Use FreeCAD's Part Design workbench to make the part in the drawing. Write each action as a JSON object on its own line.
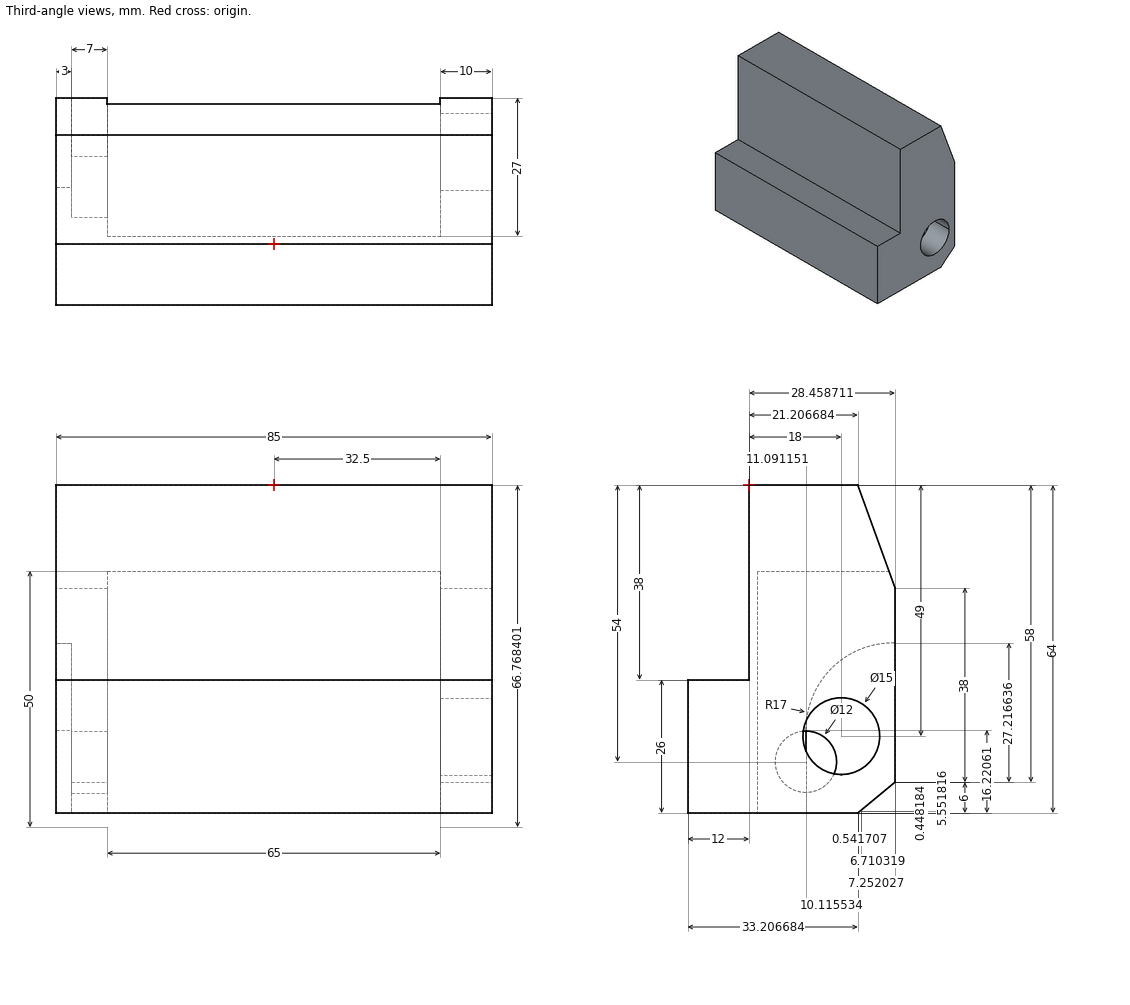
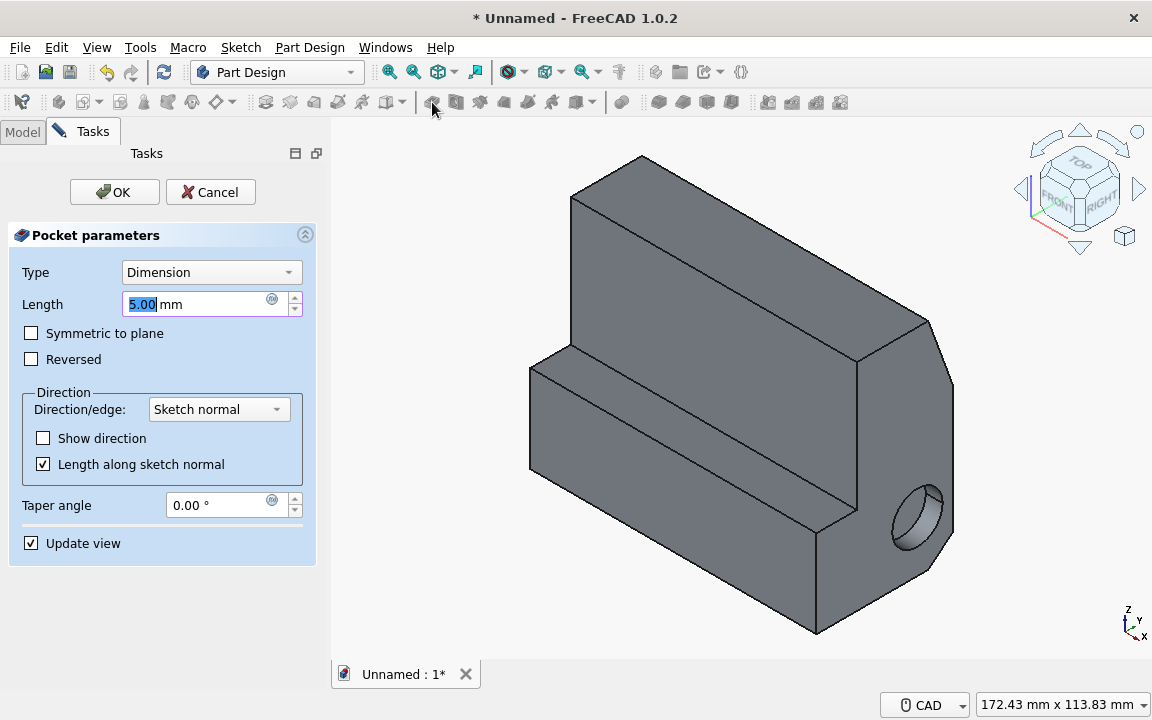
{"action": "type", "text": "10"}
{"action": "key", "text": "Tab"}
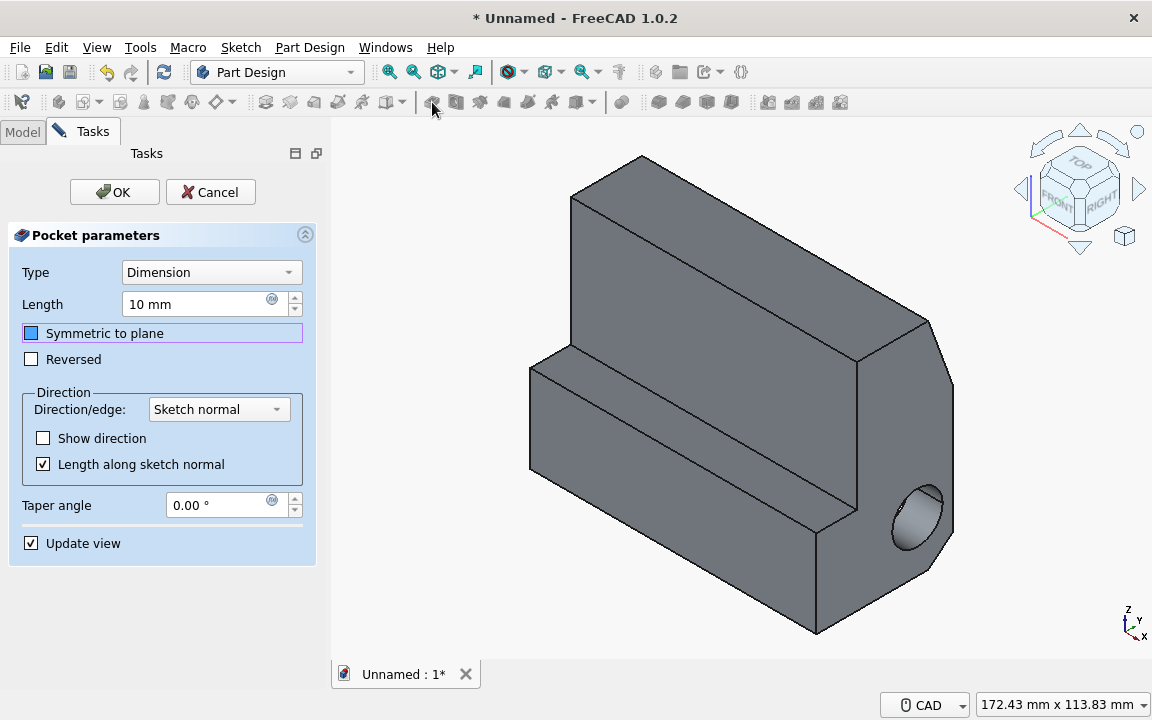
{"action": "left_click", "coordinate": [115, 192]}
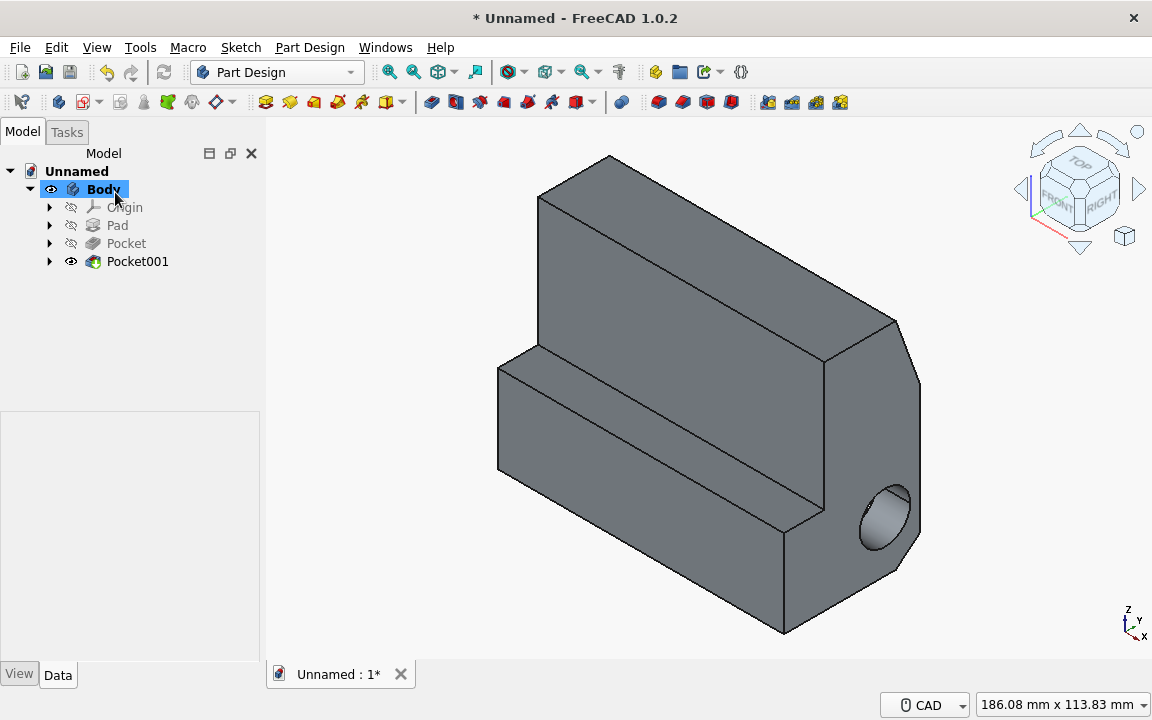
{"action": "key", "text": "6"}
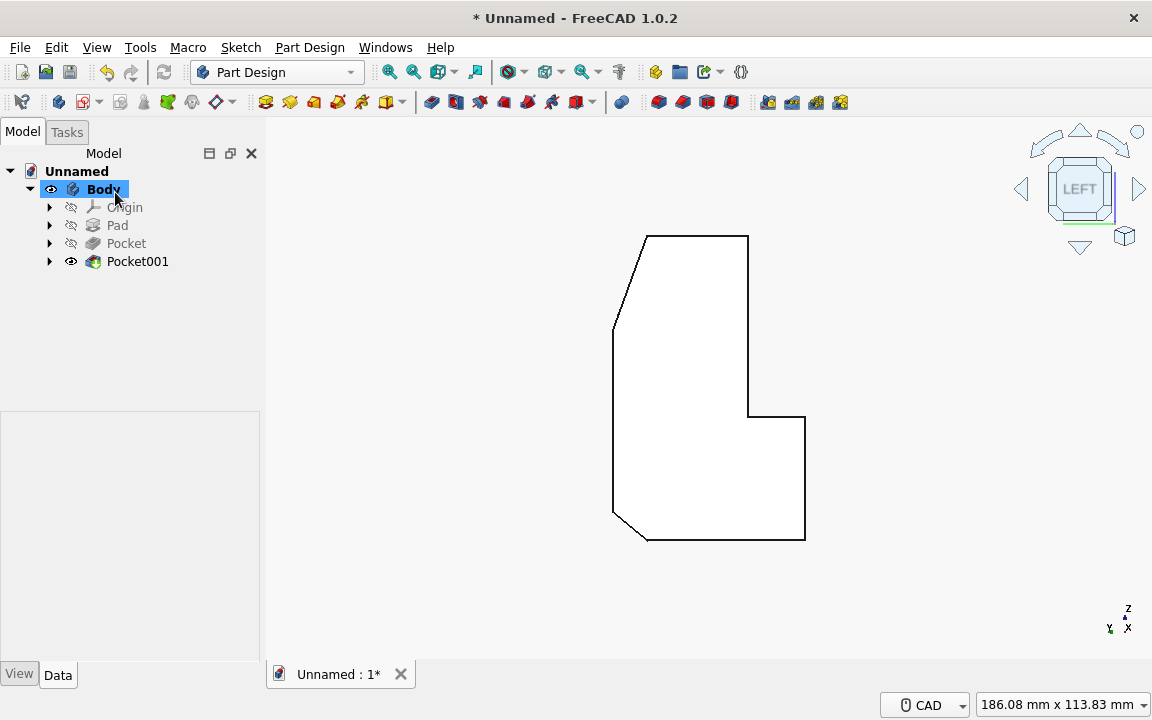
{"action": "left_click", "coordinate": [681, 431]}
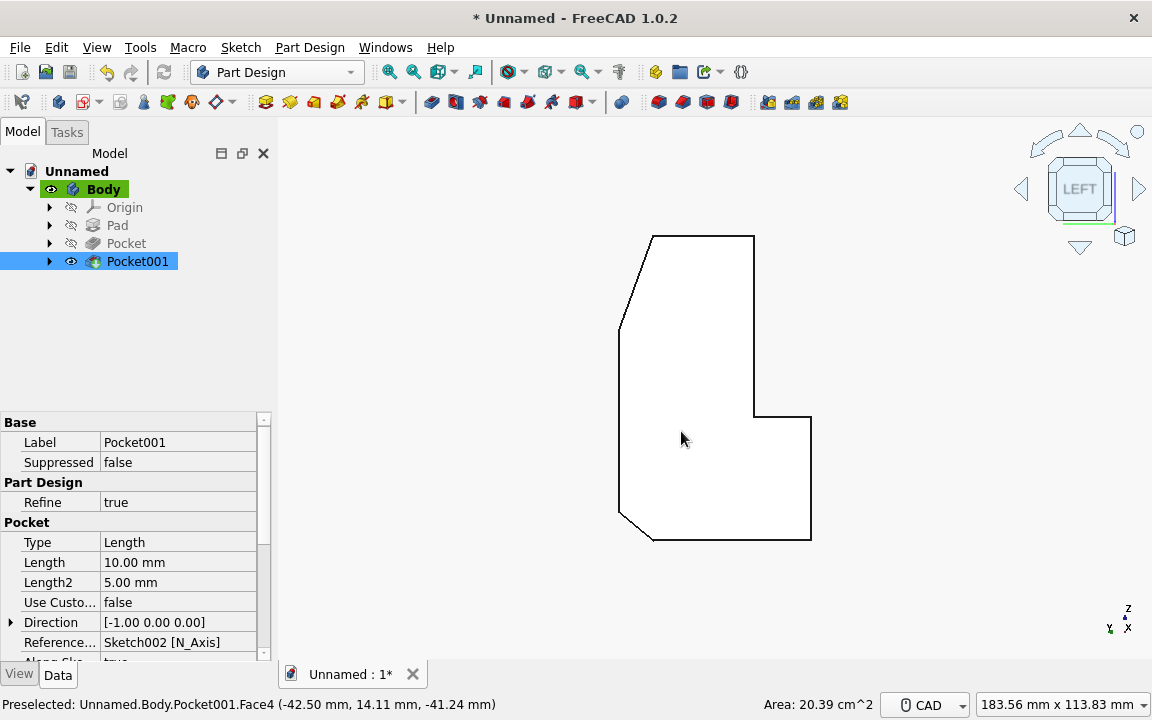
{"action": "left_click", "coordinate": [84, 102]}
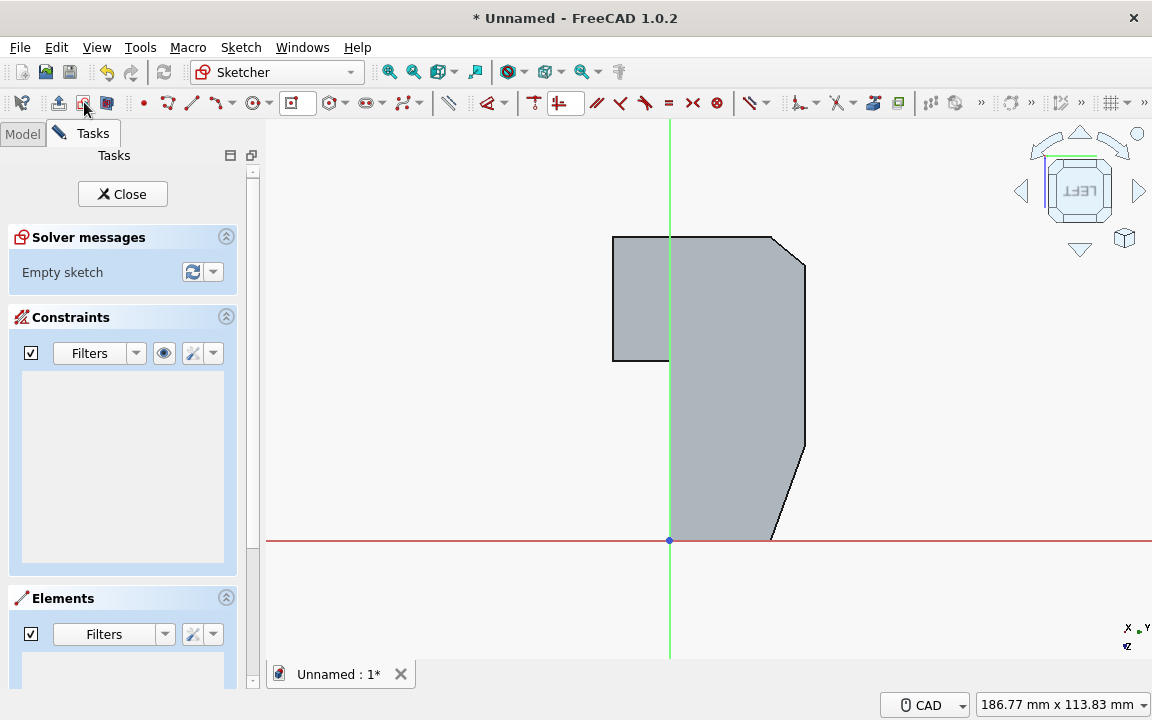
{"action": "left_click", "coordinate": [168, 104]}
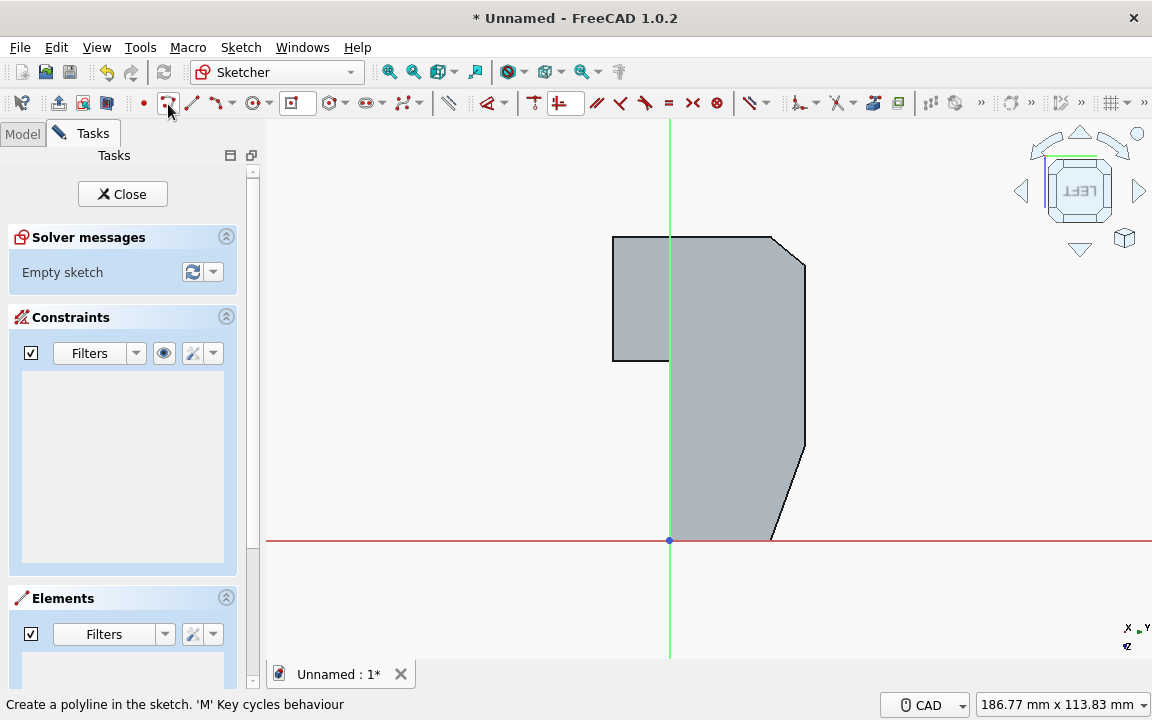
{"action": "left_click", "coordinate": [805, 395]}
{"action": "left_click", "coordinate": [805, 266]}
{"action": "left_click", "coordinate": [773, 239]}
{"action": "right_click", "coordinate": [773, 239]}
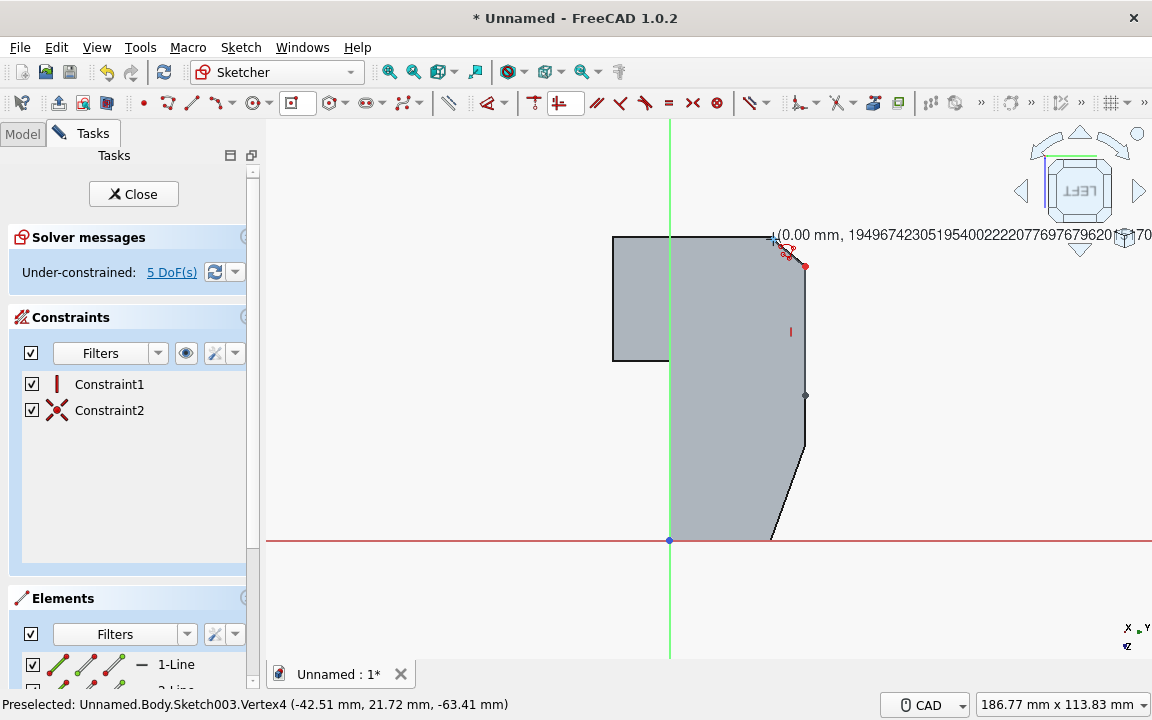
{"action": "left_click", "coordinate": [216, 104]}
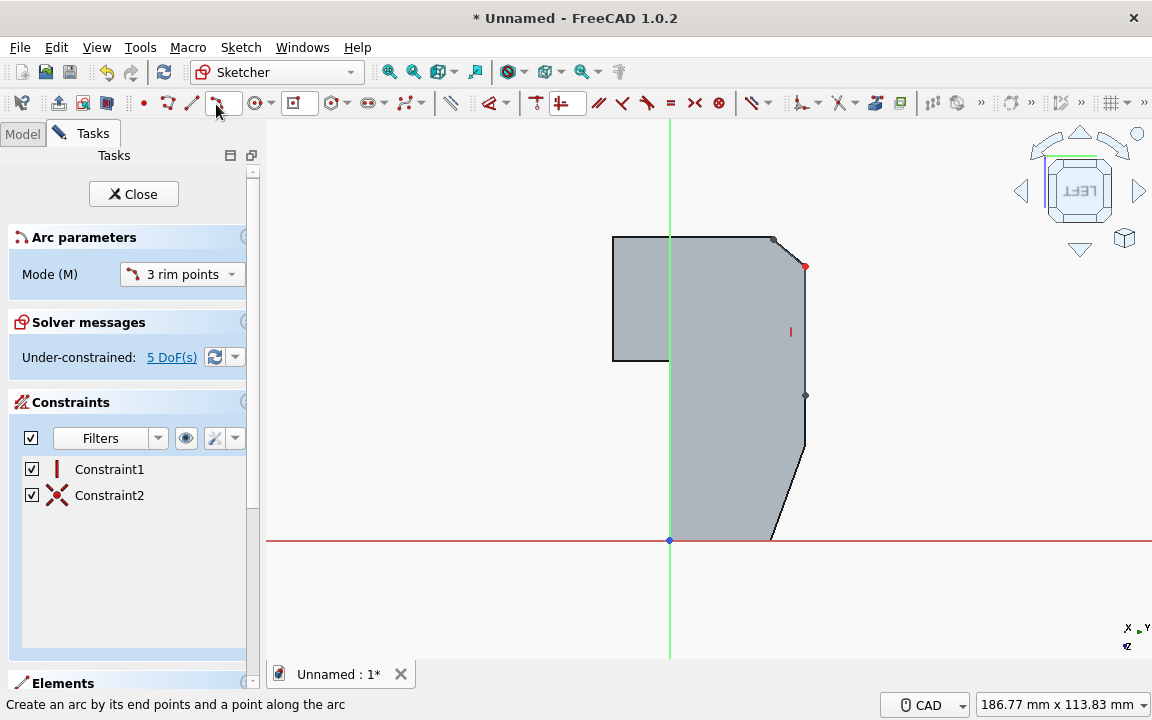
{"action": "left_click", "coordinate": [773, 240]}
{"action": "left_click", "coordinate": [805, 396]}
{"action": "left_click", "coordinate": [724, 330]}
{"action": "key", "text": "Escape"}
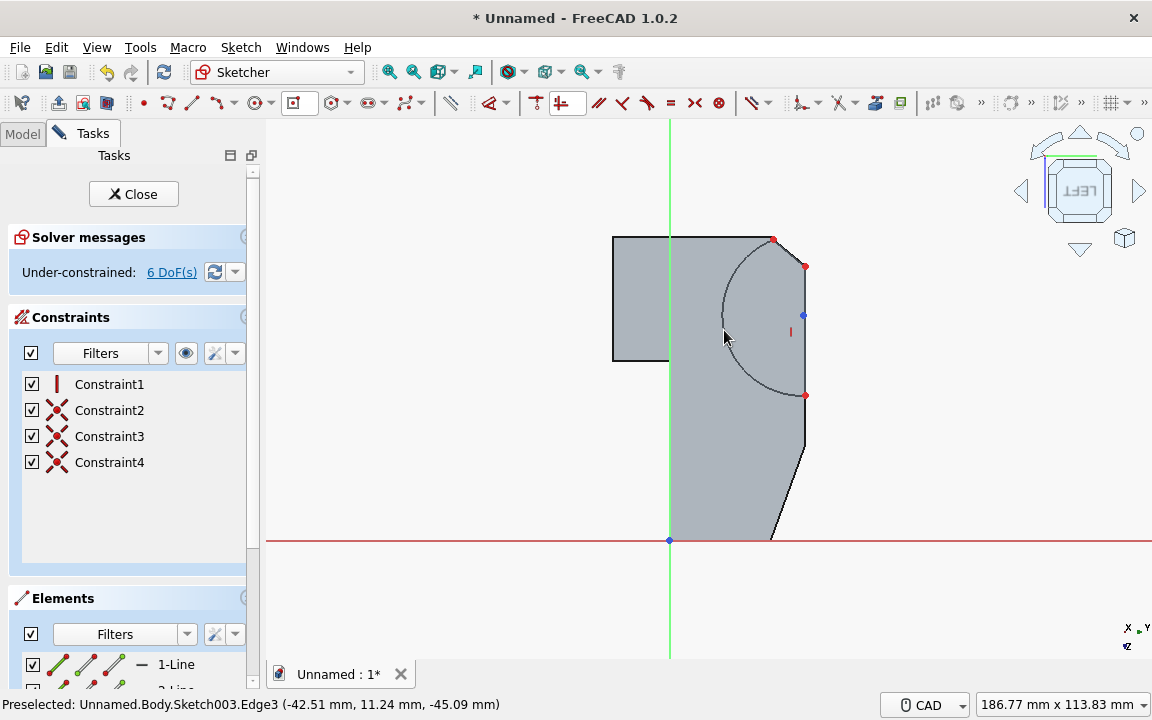
{"action": "left_click", "coordinate": [490, 104]}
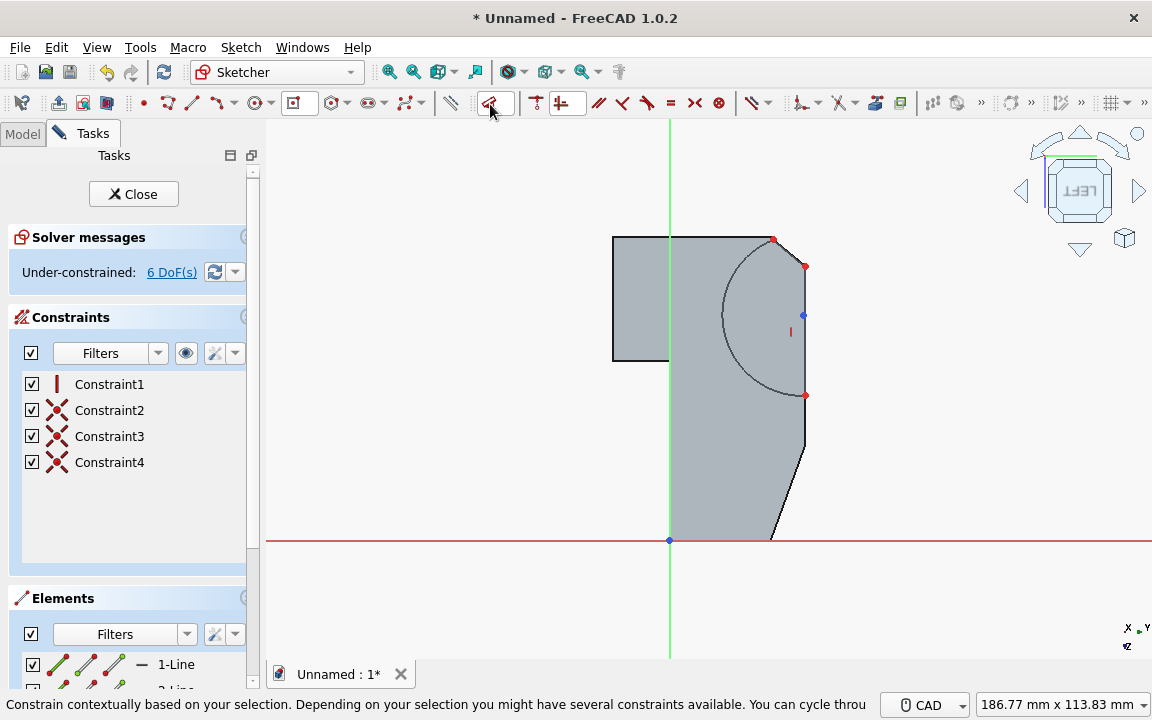
{"action": "left_click", "coordinate": [727, 287]}
{"action": "left_click", "coordinate": [697, 276]}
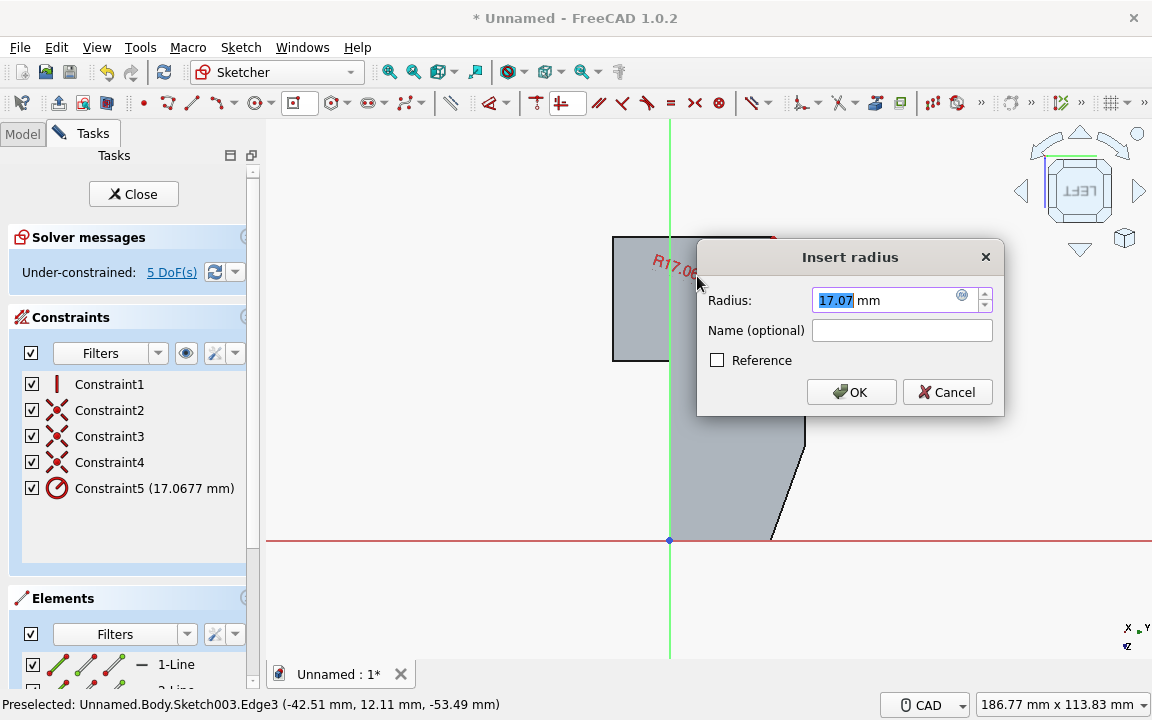
{"action": "type", "text": "17"}
{"action": "key", "text": "Return"}